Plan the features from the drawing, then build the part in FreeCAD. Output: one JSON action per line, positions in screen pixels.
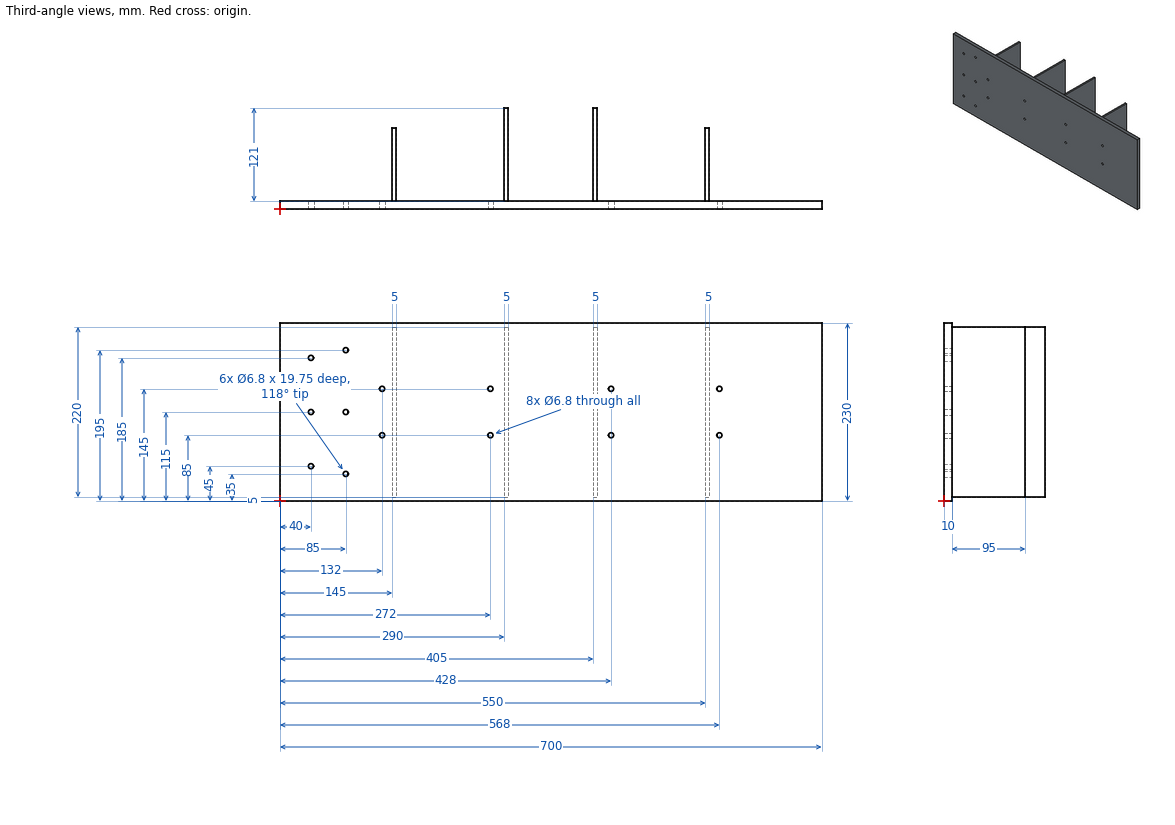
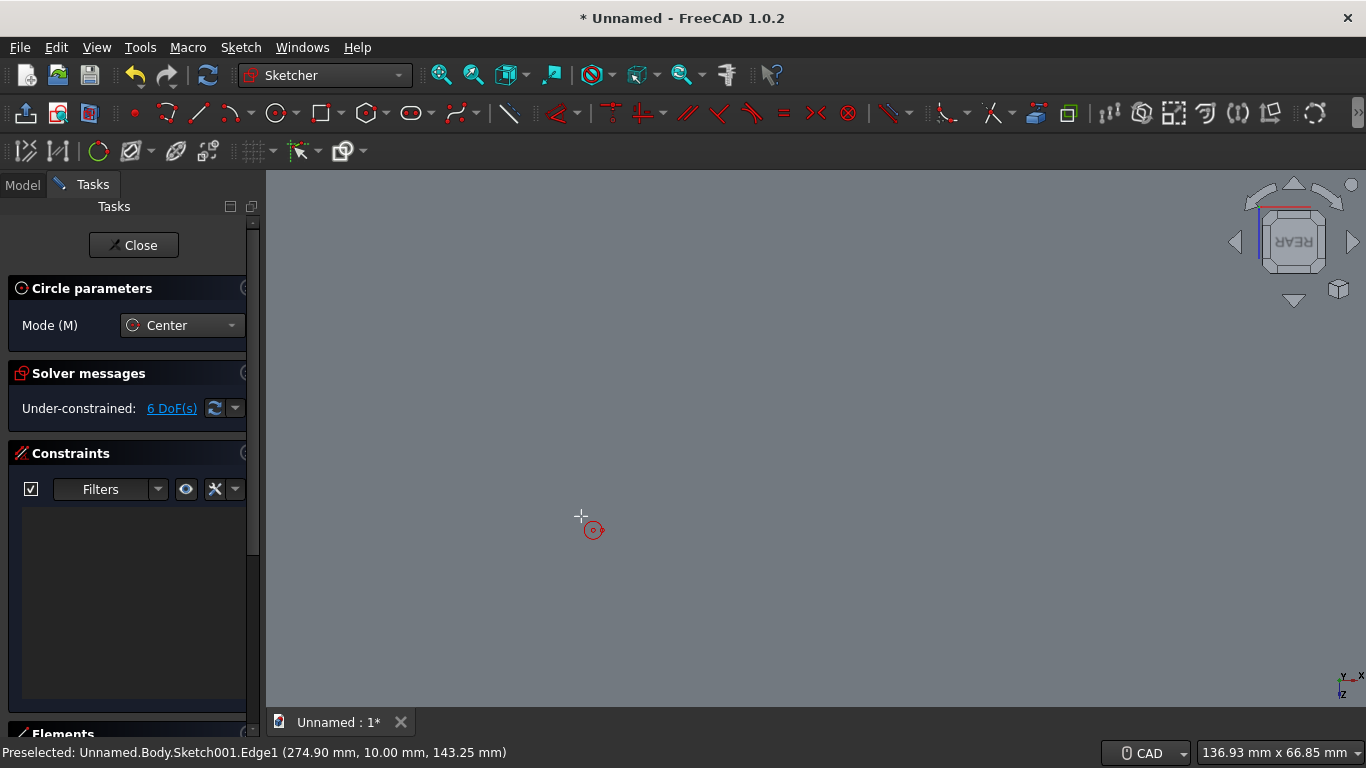
{"action": "scroll", "coordinate": [580, 517], "scroll_direction": "down", "scroll_amount": 10}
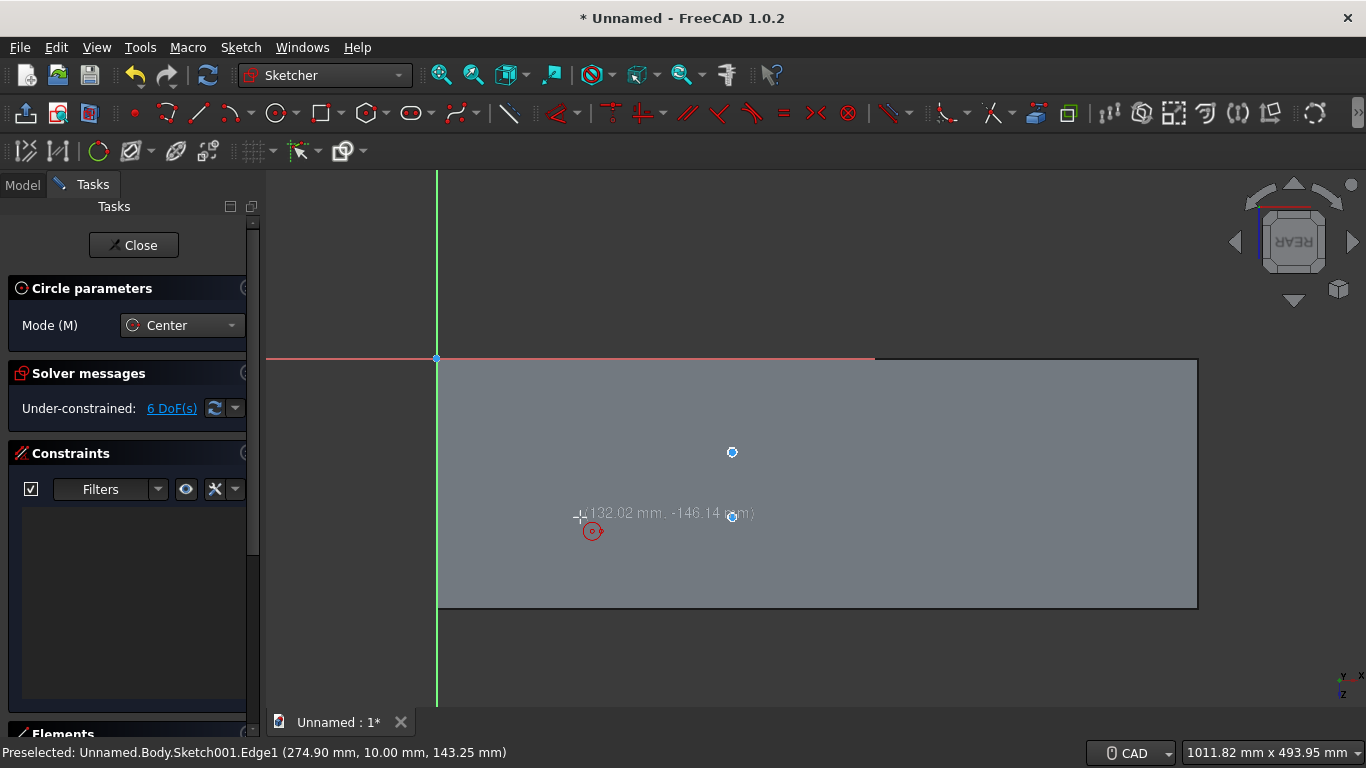
{"action": "left_click", "coordinate": [580, 516]}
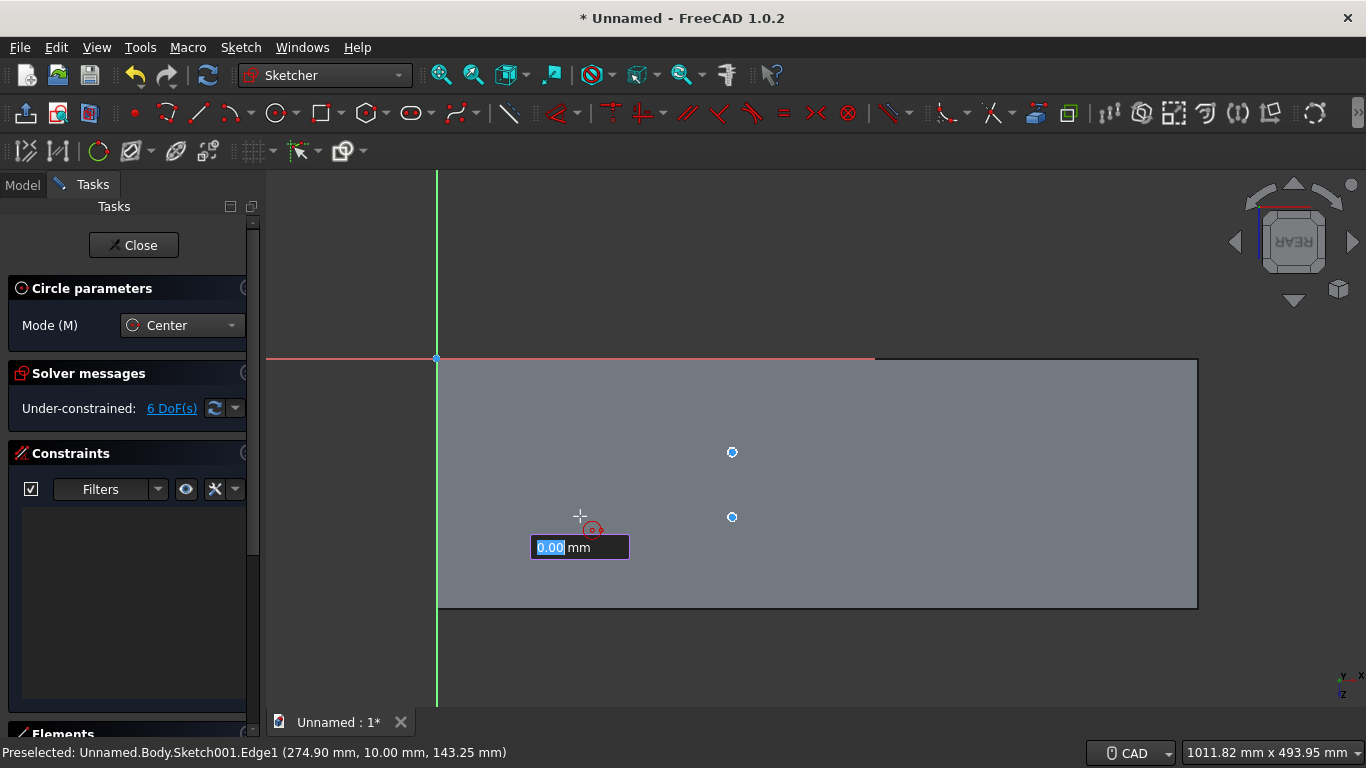
{"action": "scroll", "coordinate": [583, 514], "scroll_direction": "up", "scroll_amount": 8}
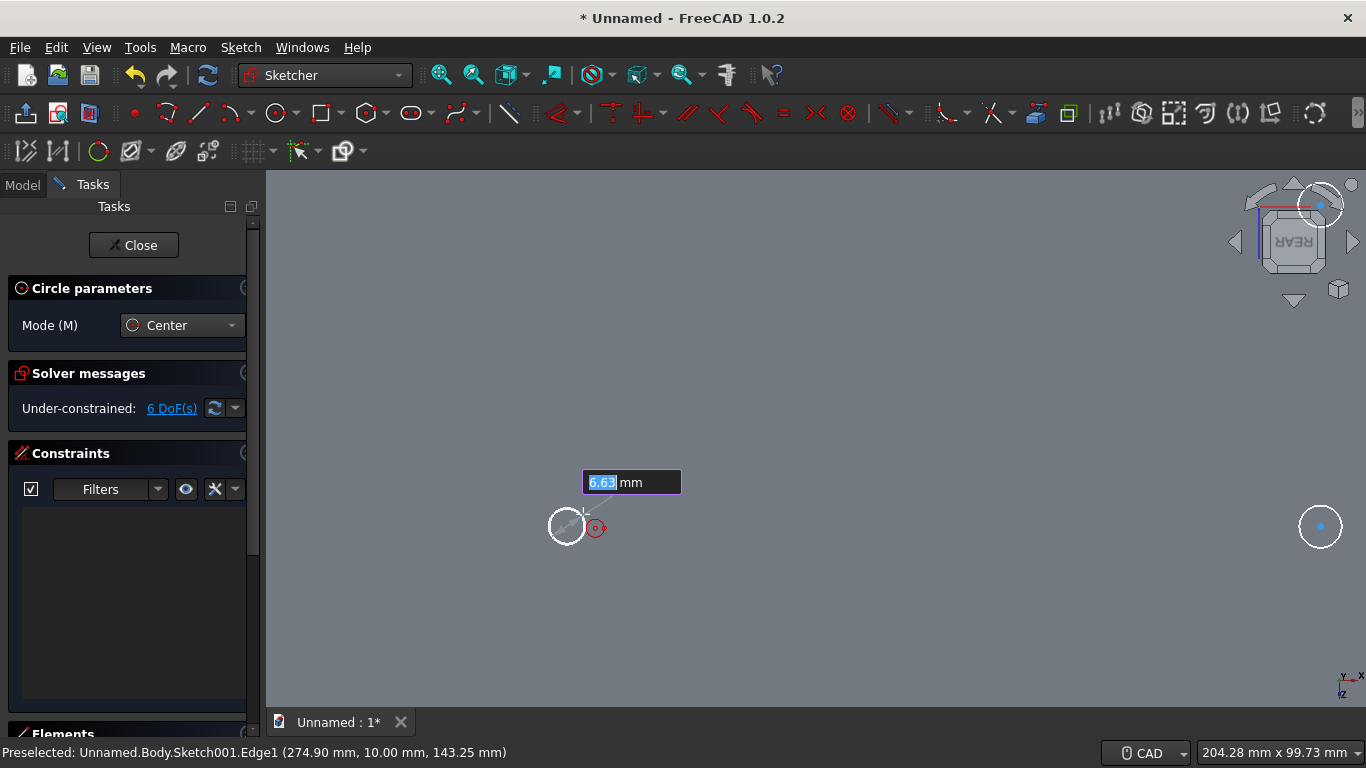
{"action": "left_click", "coordinate": [581, 511]}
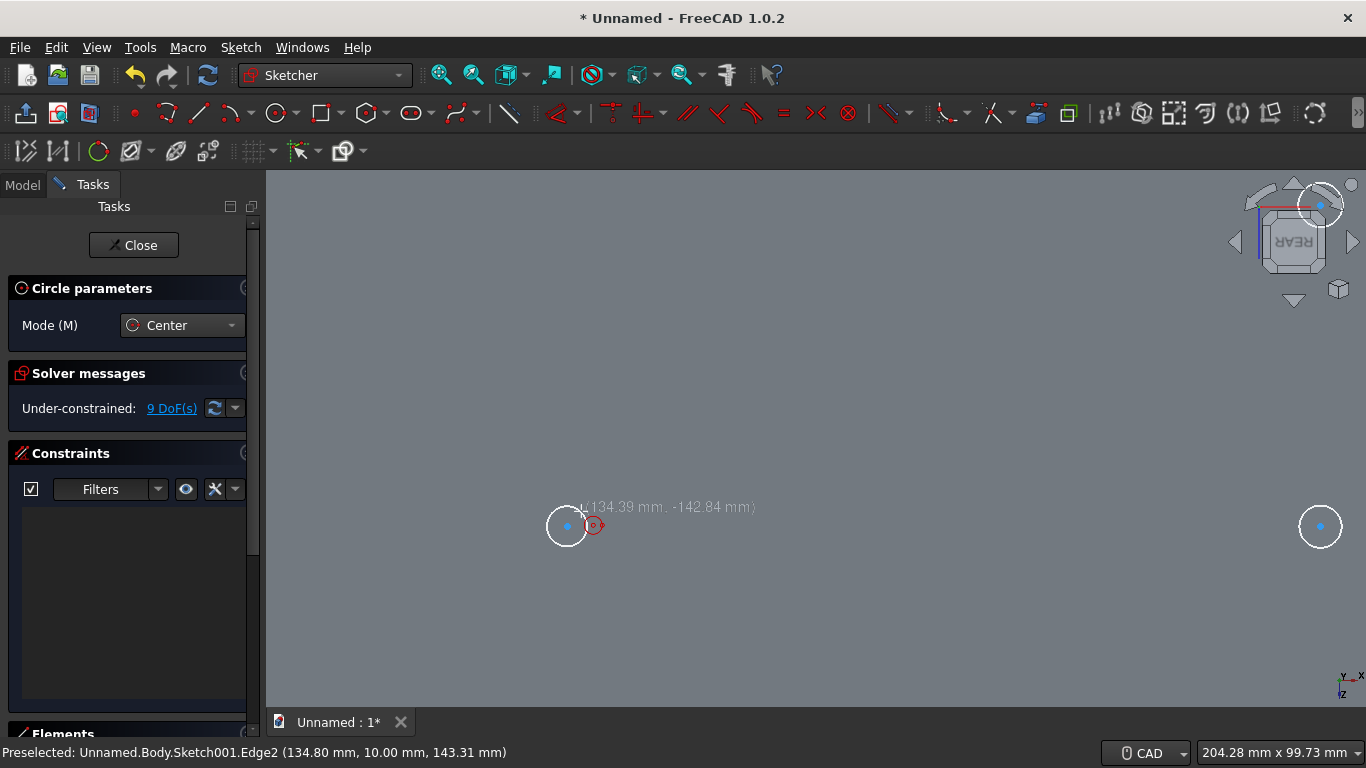
{"action": "scroll", "coordinate": [568, 201], "scroll_direction": "up", "scroll_amount": 2}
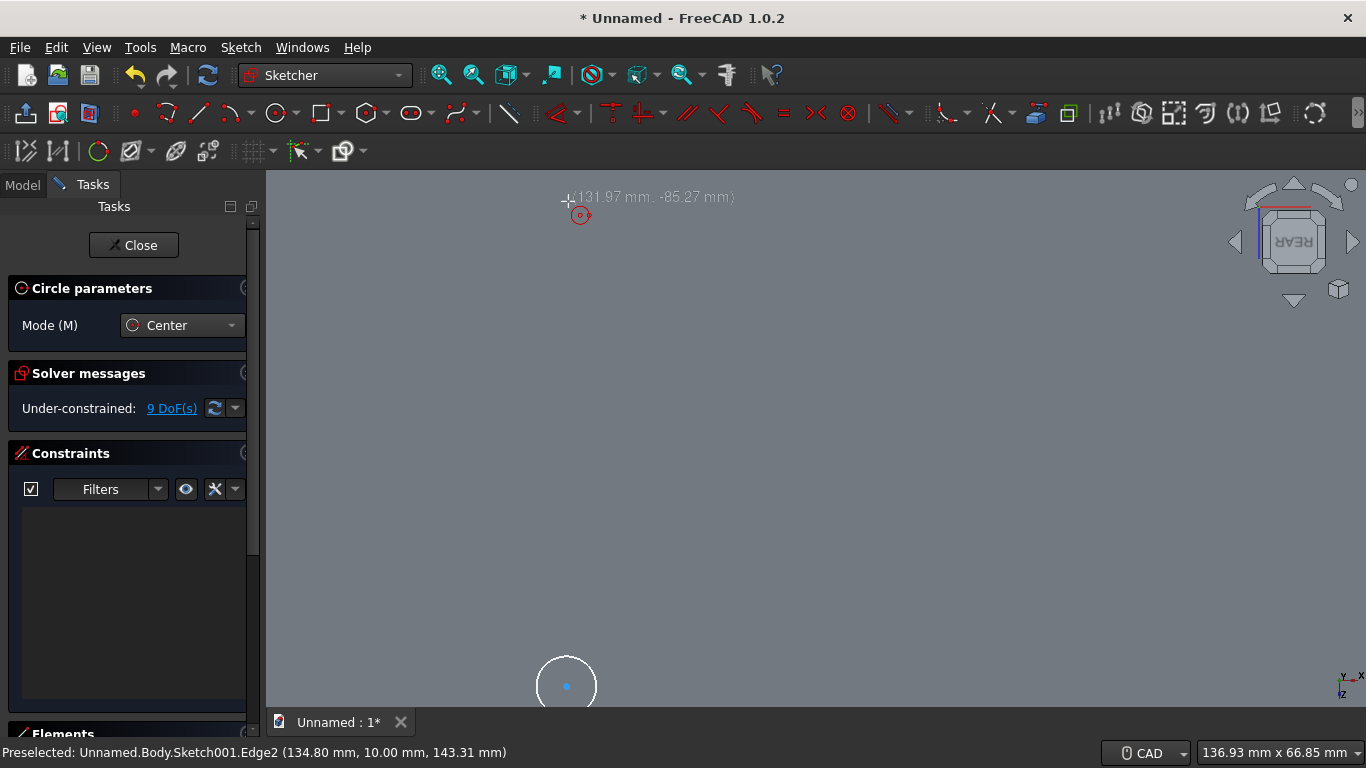
{"action": "scroll", "coordinate": [582, 489], "scroll_direction": "down", "scroll_amount": 10}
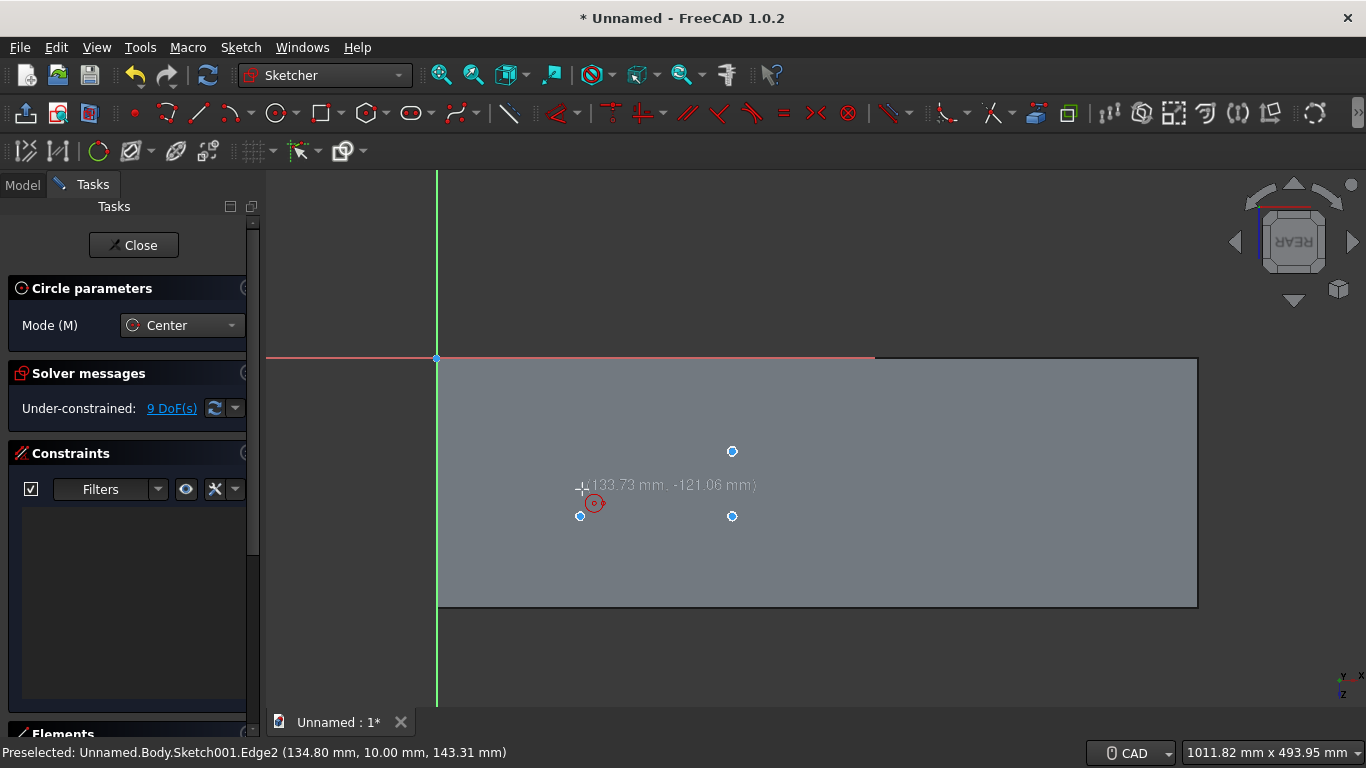
{"action": "left_click", "coordinate": [580, 450]}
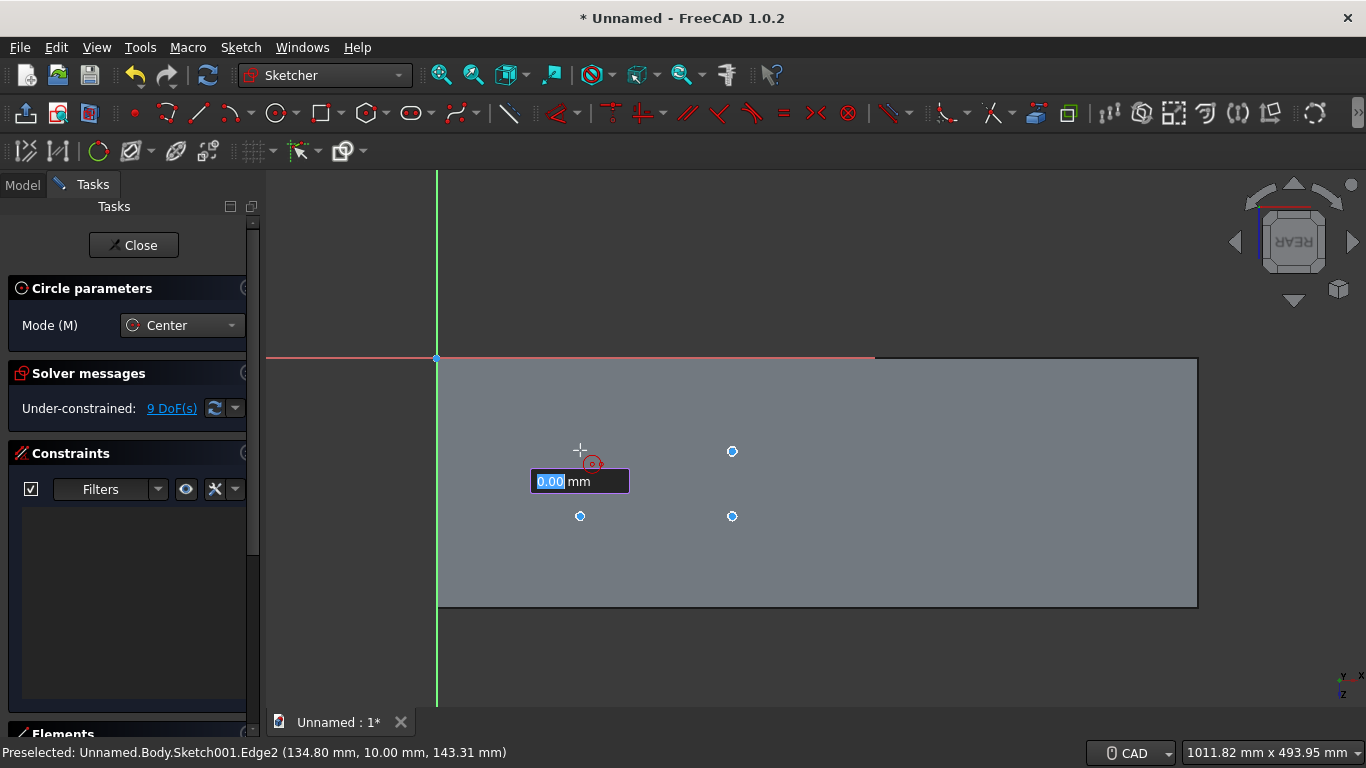
{"action": "scroll", "coordinate": [583, 448], "scroll_direction": "up", "scroll_amount": 8}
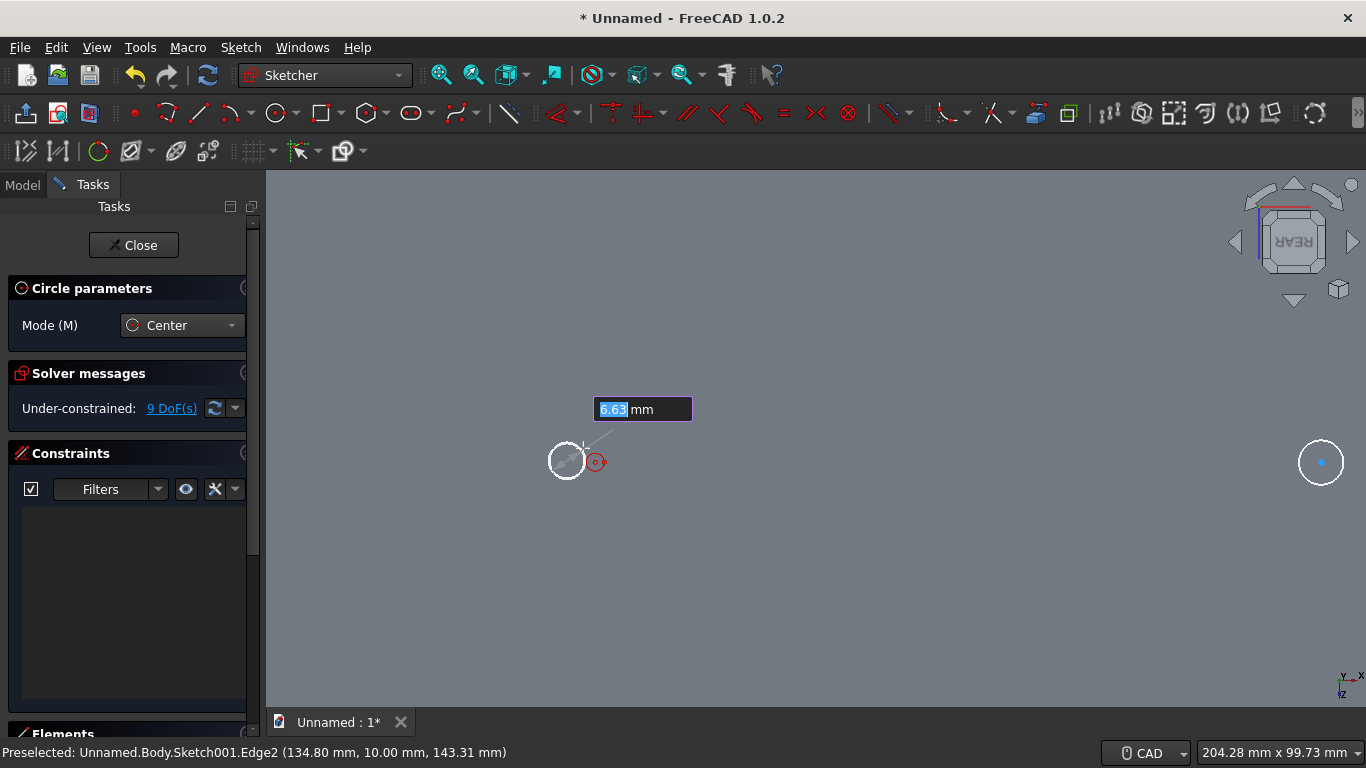
{"action": "left_click", "coordinate": [582, 445]}